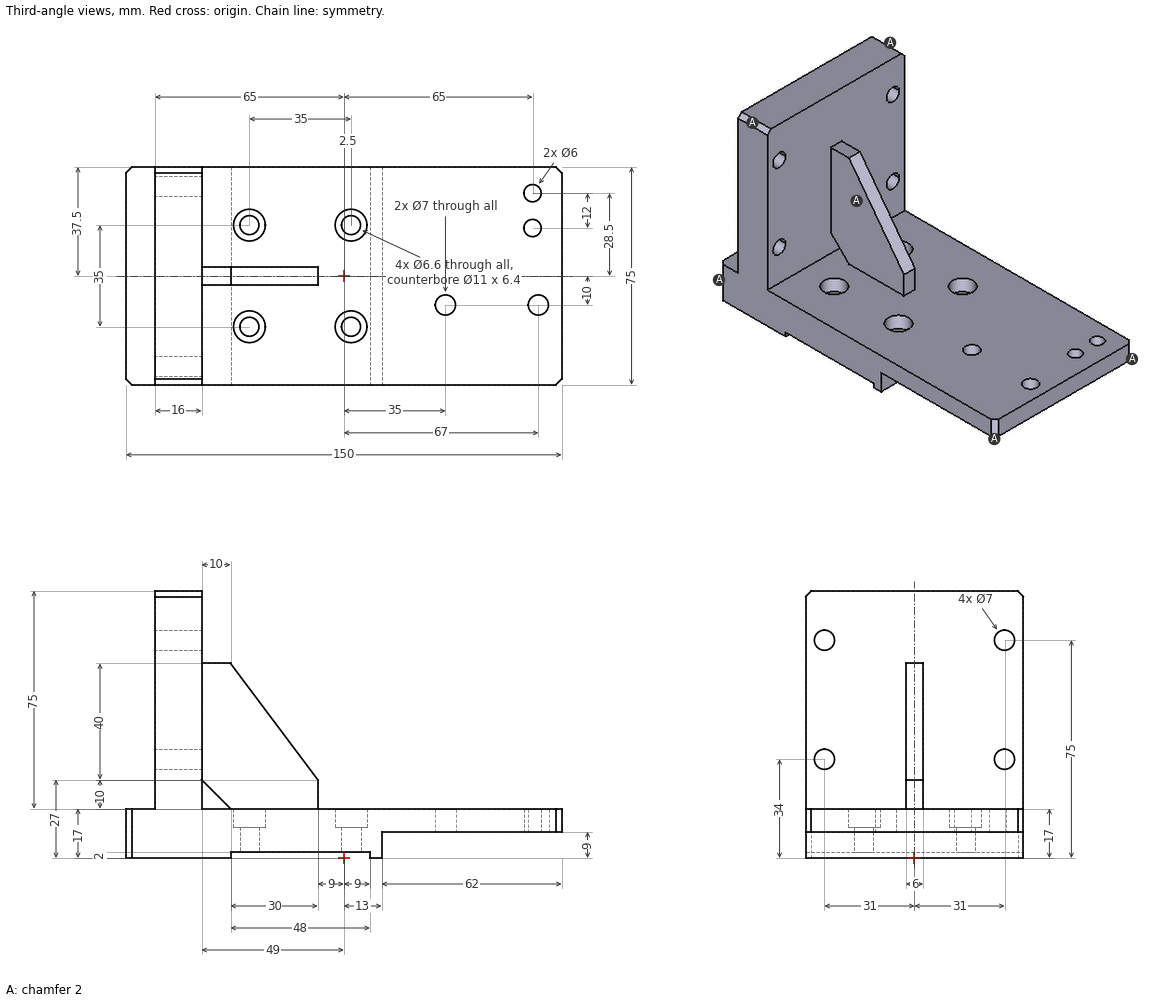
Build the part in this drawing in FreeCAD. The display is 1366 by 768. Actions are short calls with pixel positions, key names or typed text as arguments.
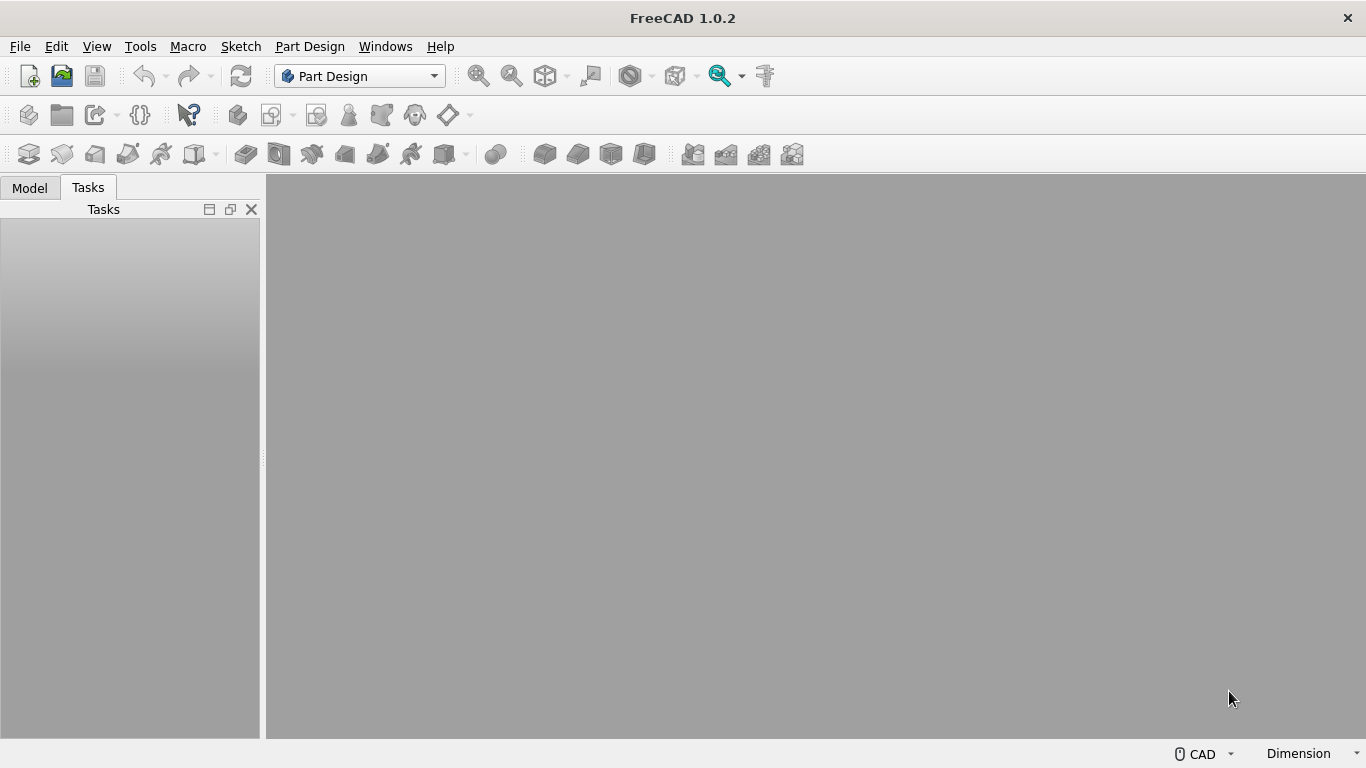
click(29, 76)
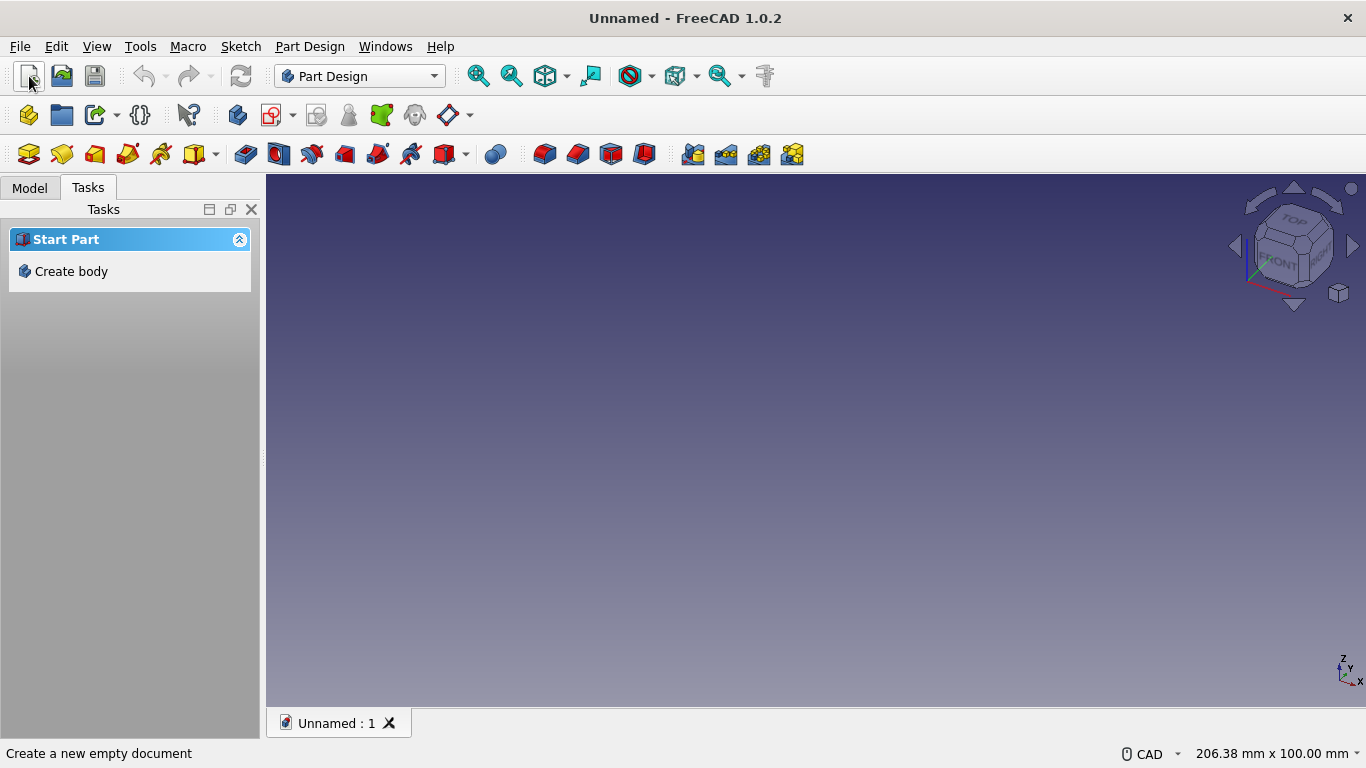
click(270, 116)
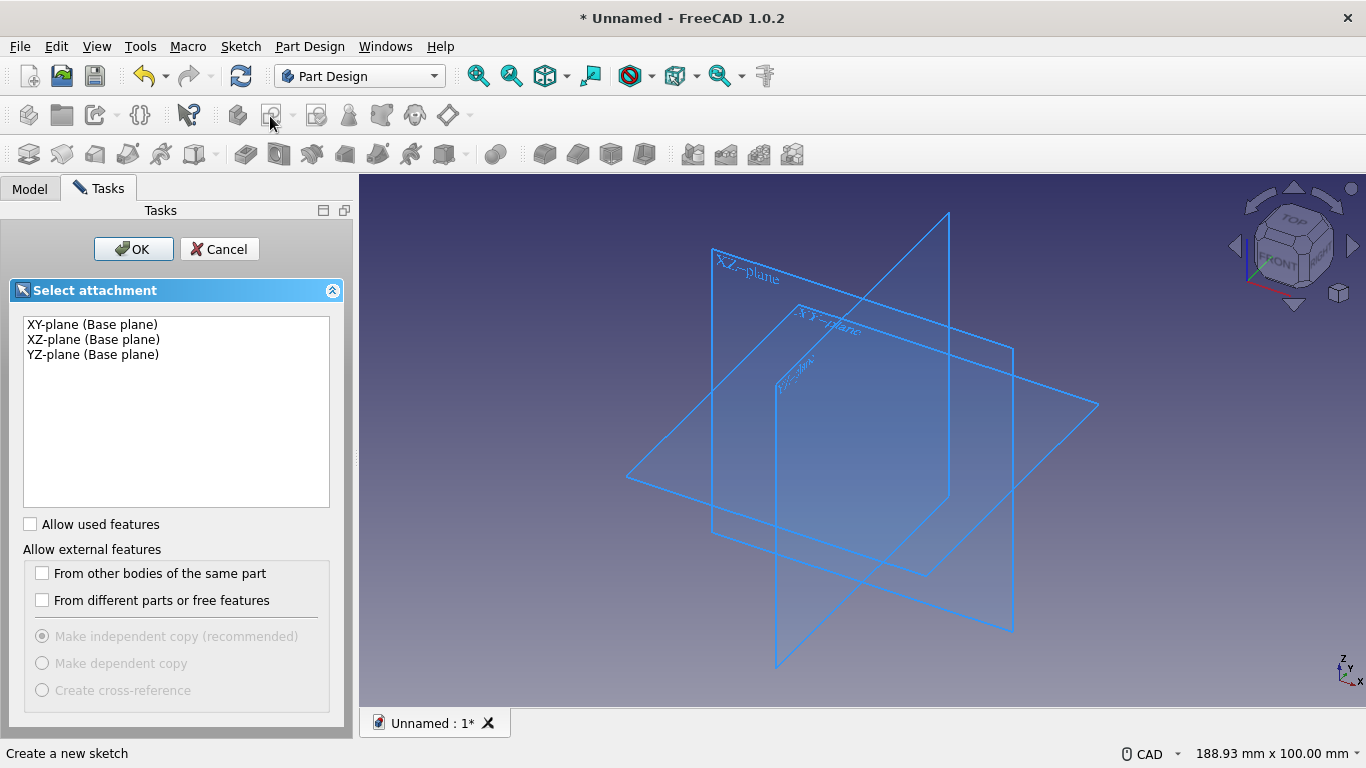
click(84, 324)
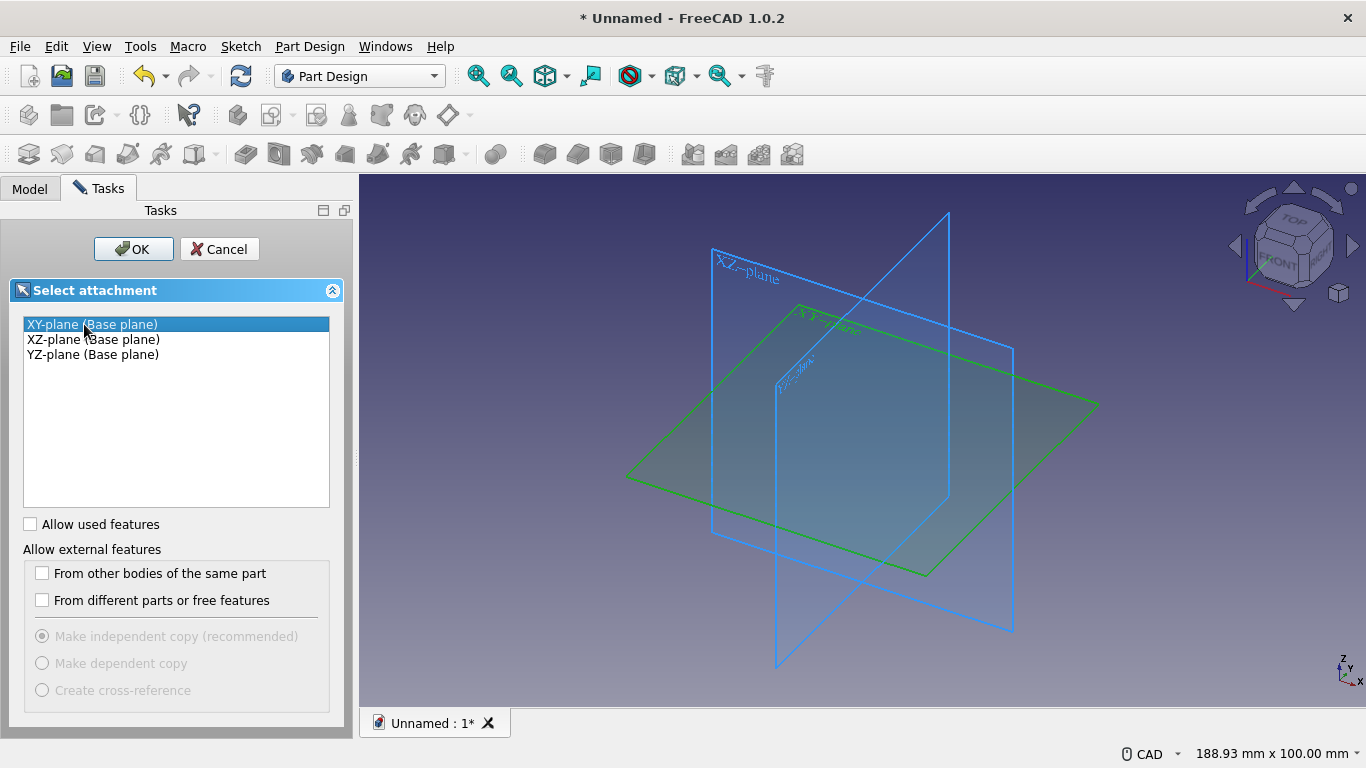
click(134, 249)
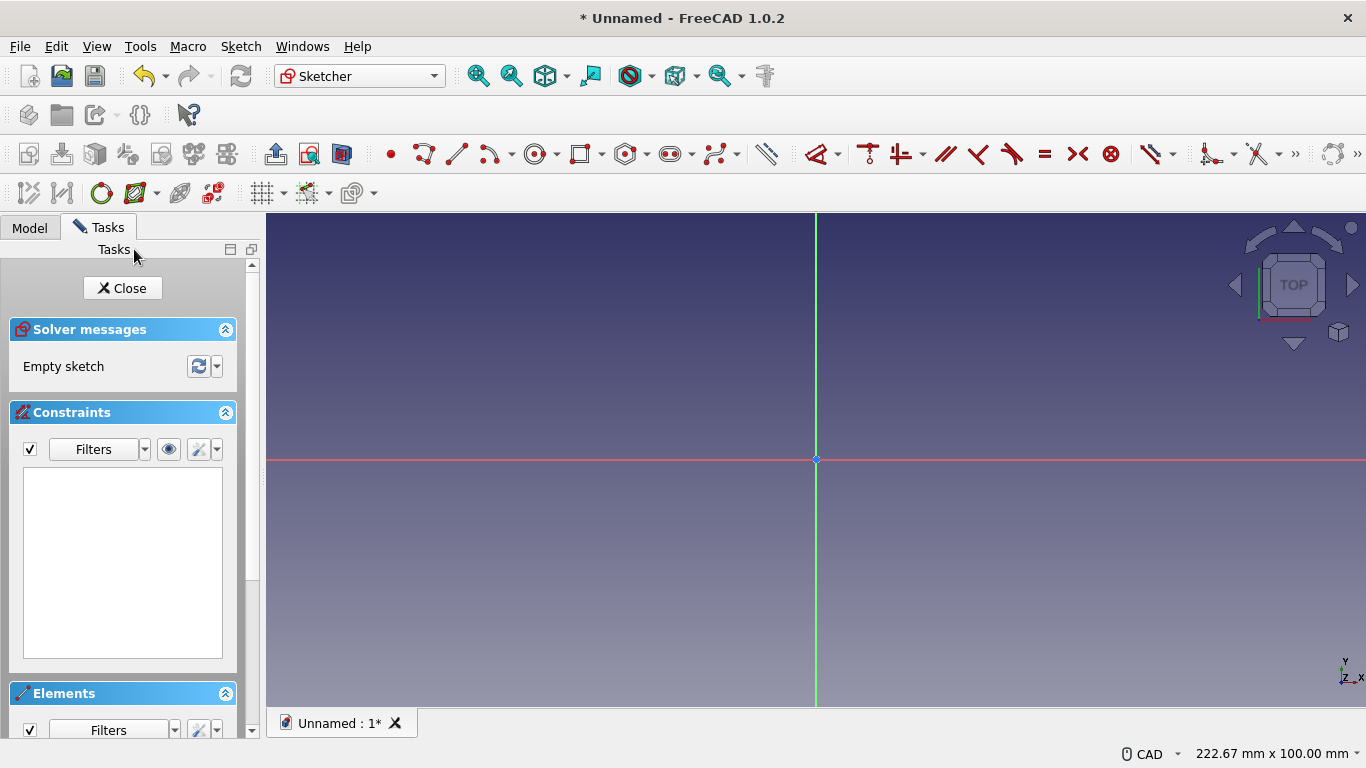
scroll(438, 460, down, 1)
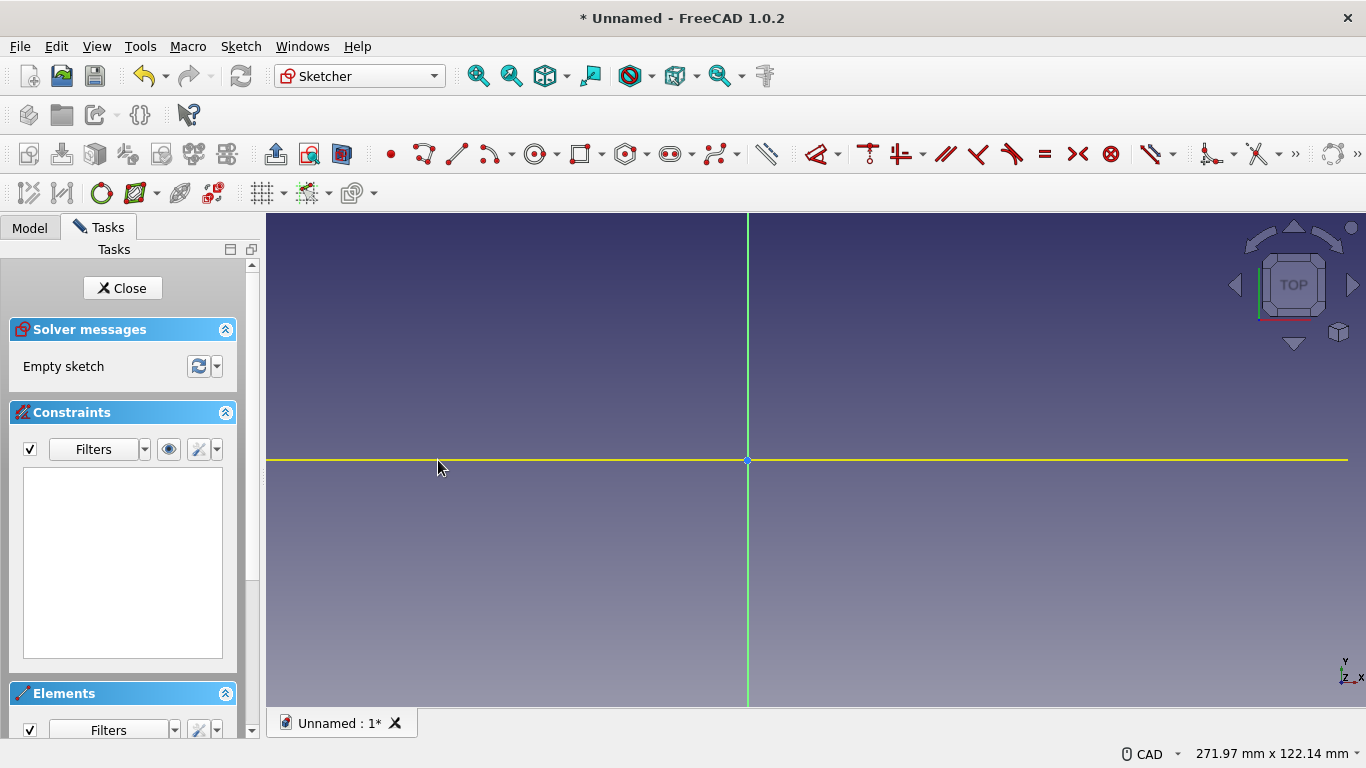
key(g)
key(v)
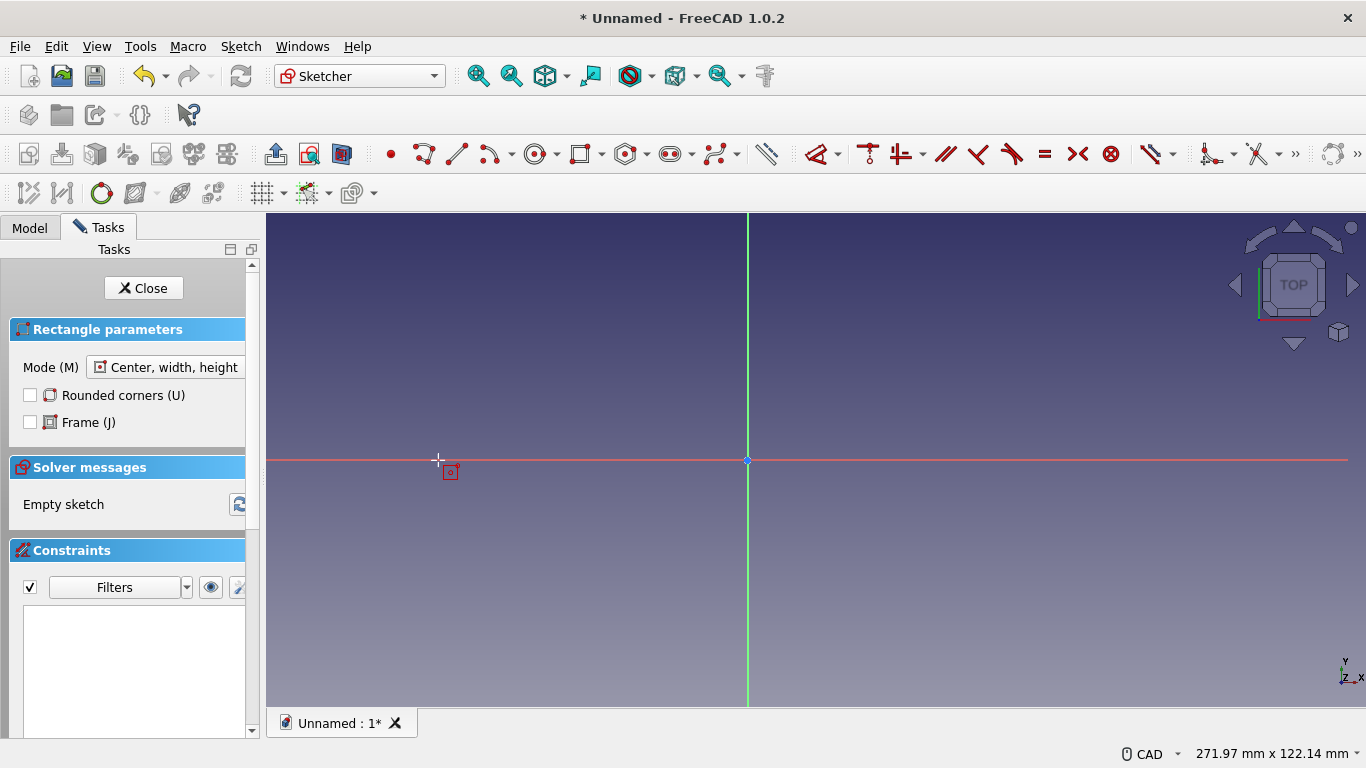
click(748, 460)
move(1051, 308)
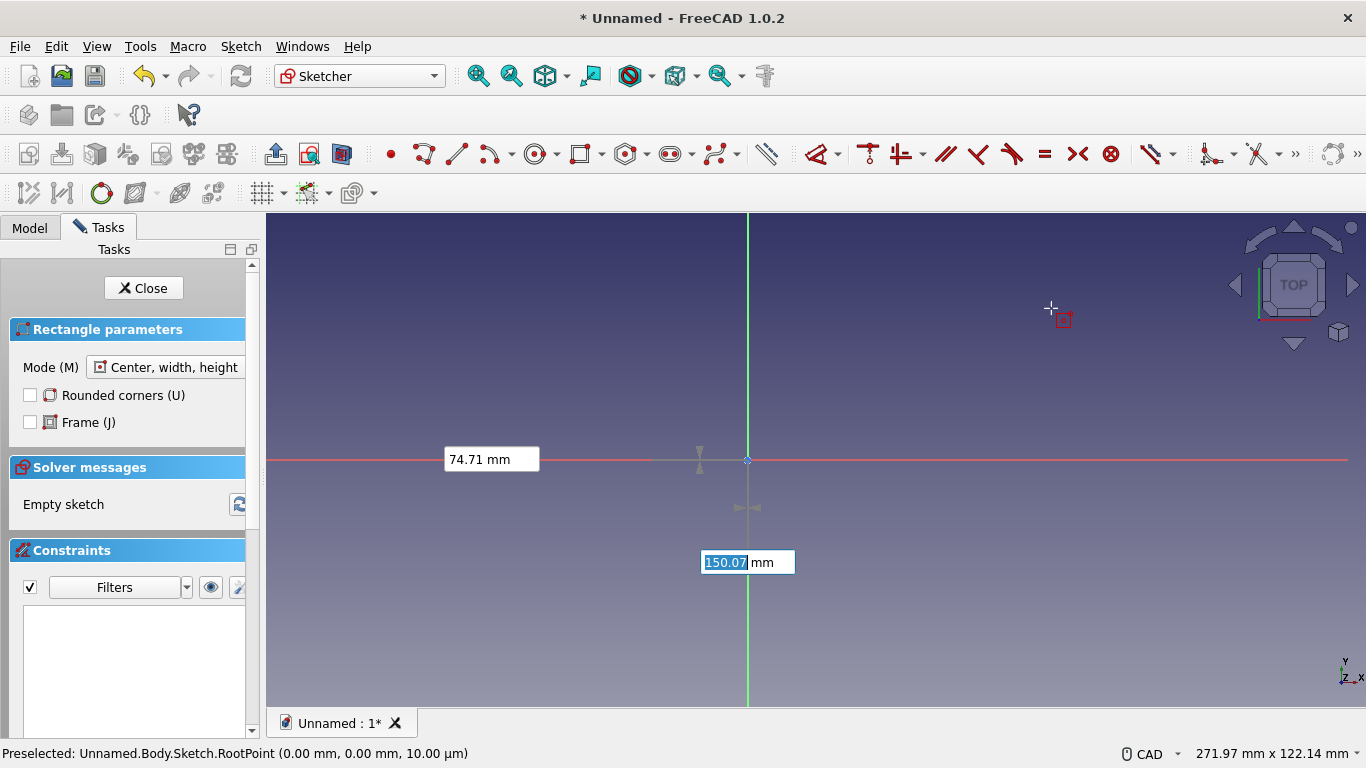
text(150)
key(Tab)
text(75)
key(Return)
key(Escape)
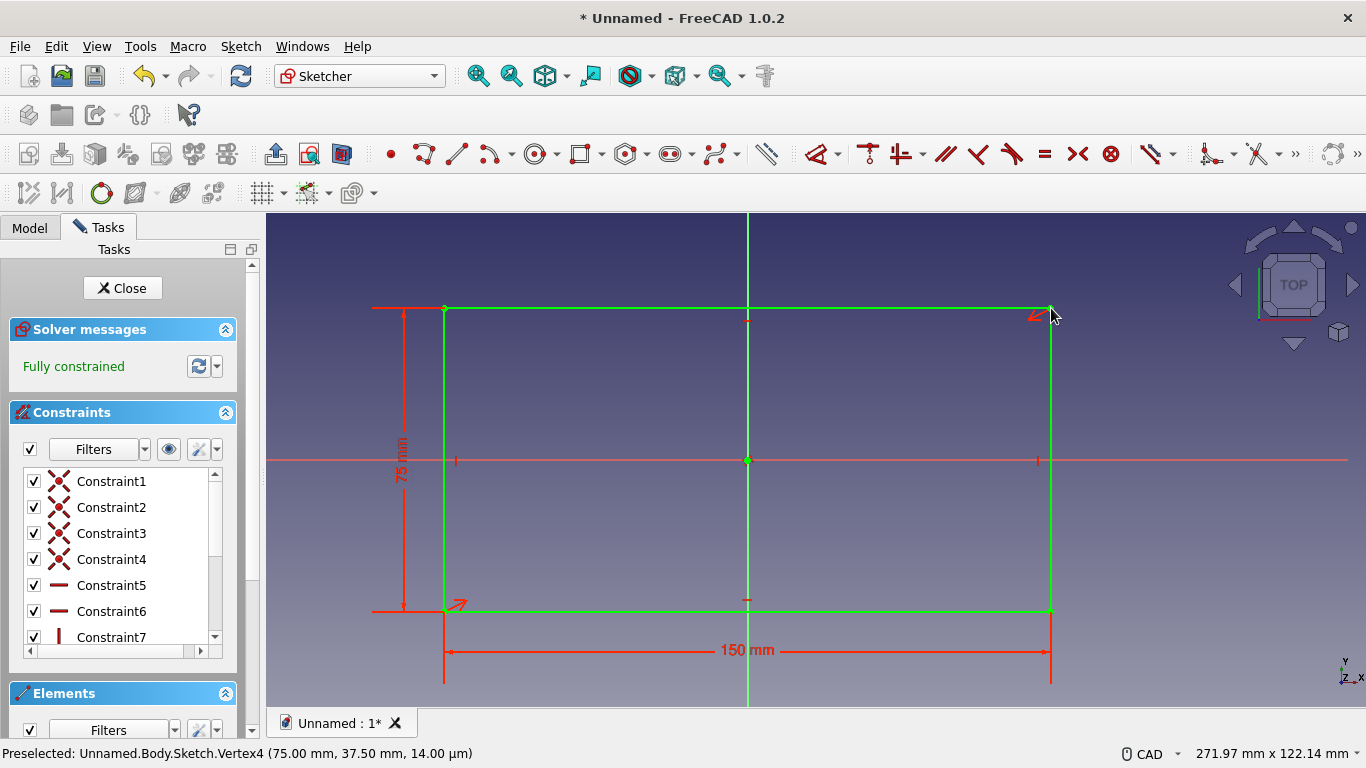
click(123, 288)